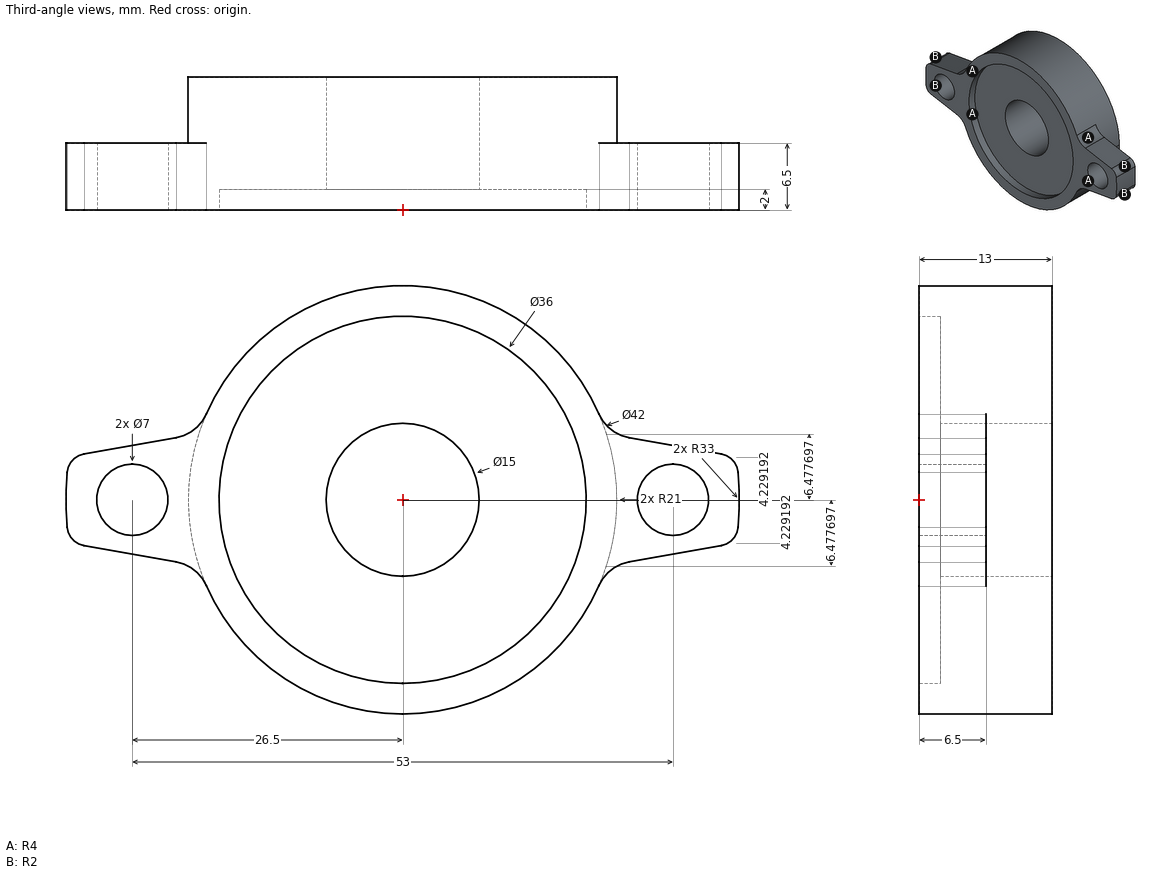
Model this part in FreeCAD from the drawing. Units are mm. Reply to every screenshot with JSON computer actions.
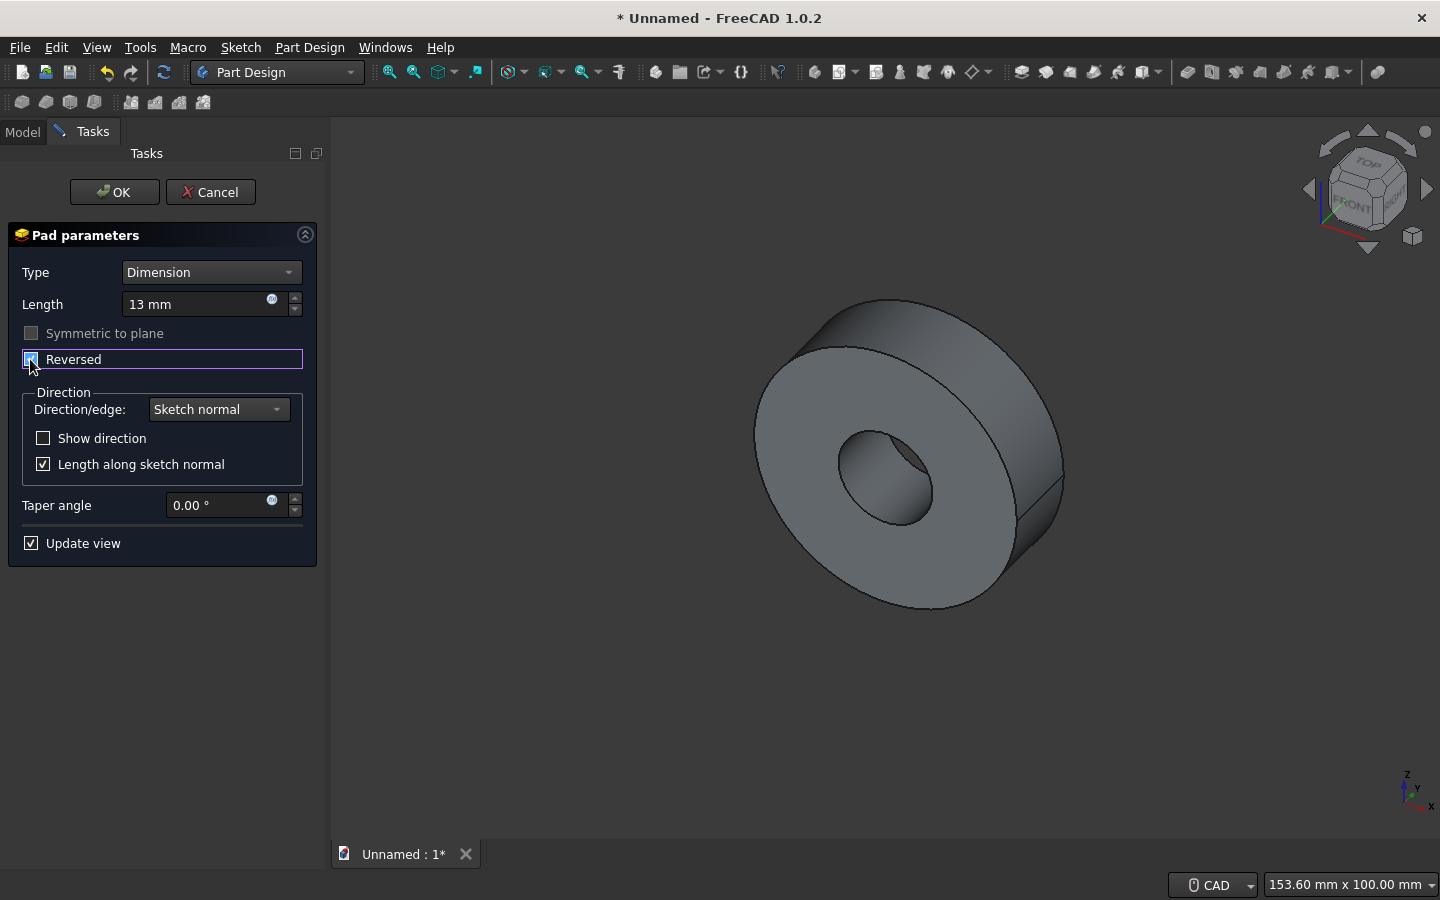
{"action": "left_click", "coordinate": [115, 192]}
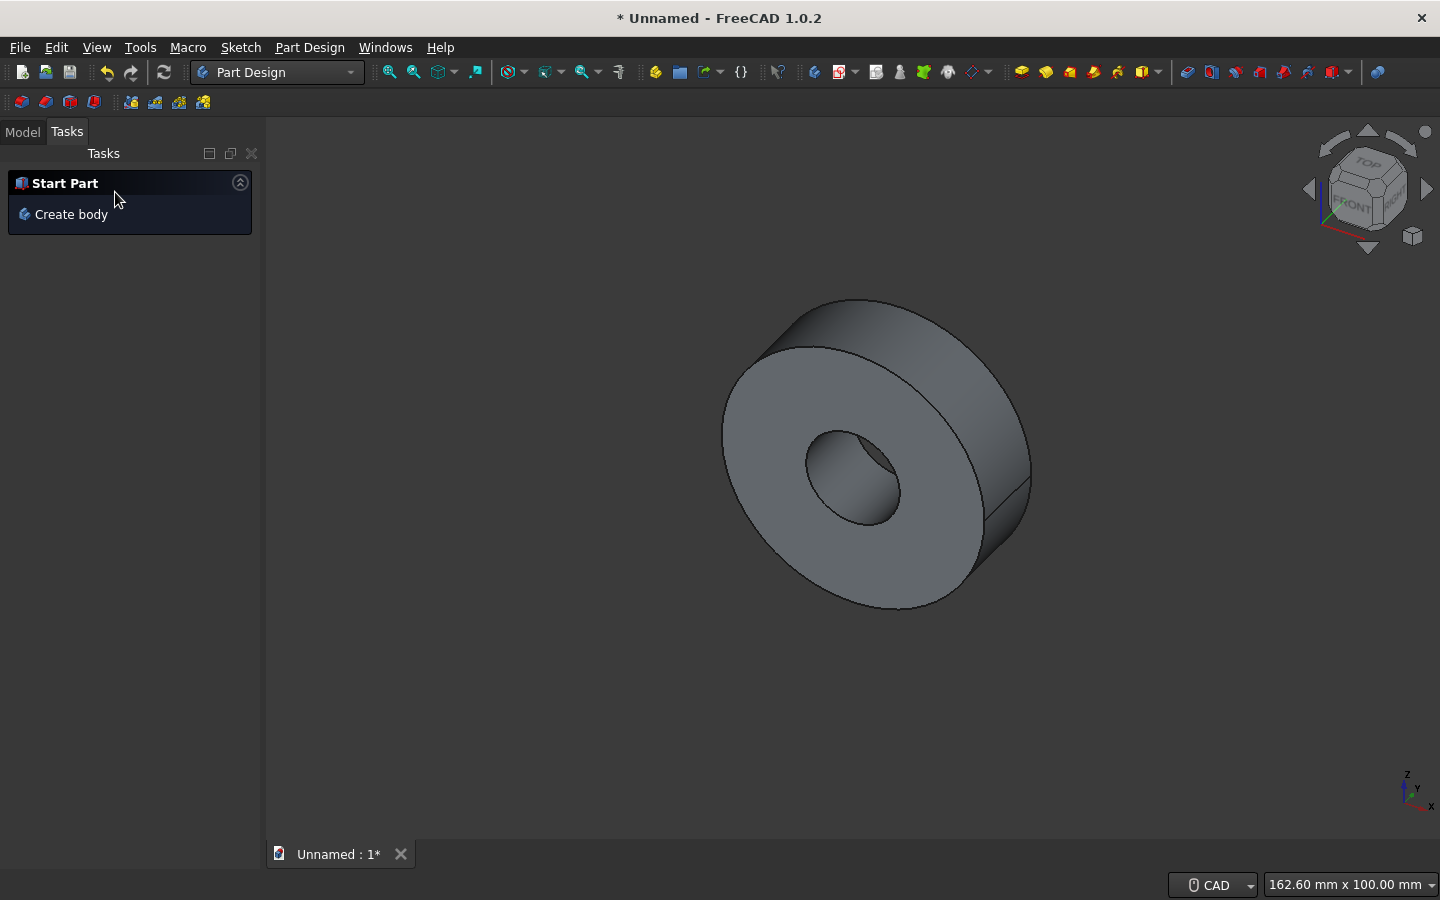
{"action": "left_click", "coordinate": [815, 536]}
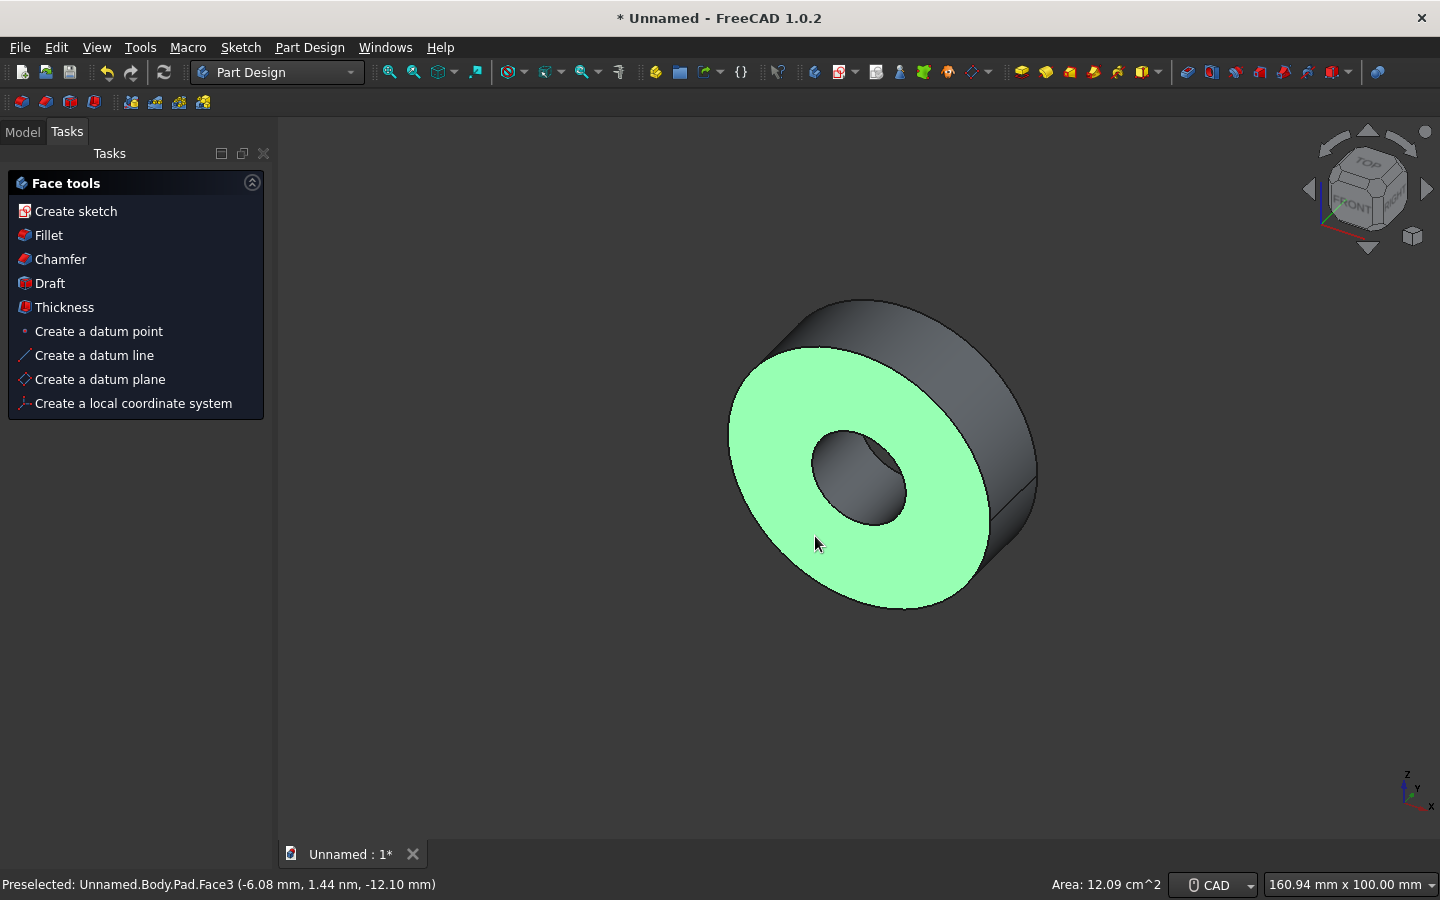
{"action": "left_click", "coordinate": [840, 72]}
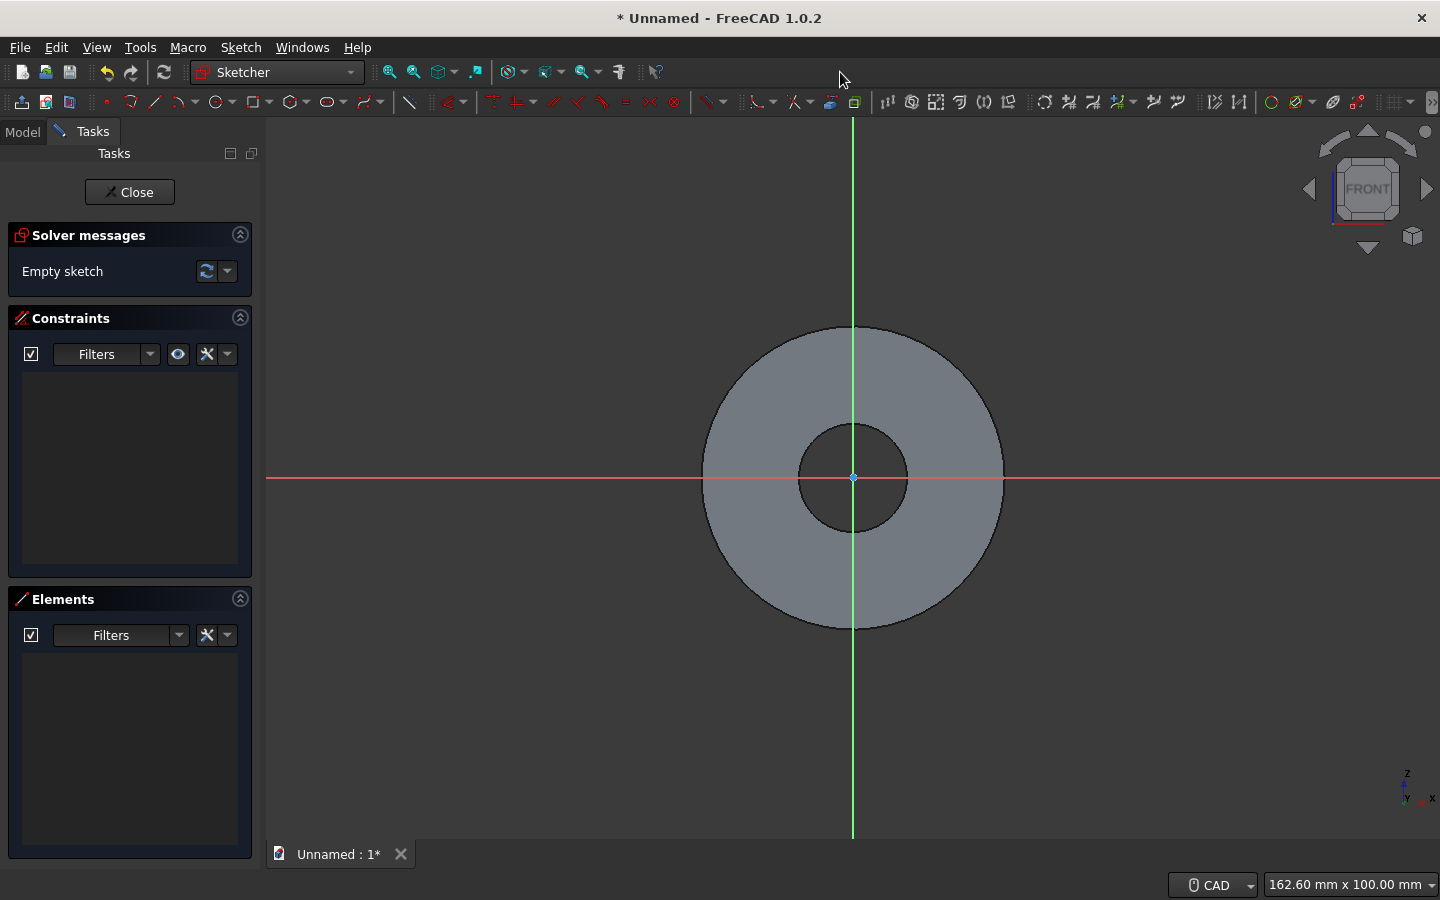
{"action": "scroll", "coordinate": [992, 478], "scroll_direction": "up", "scroll_amount": 2}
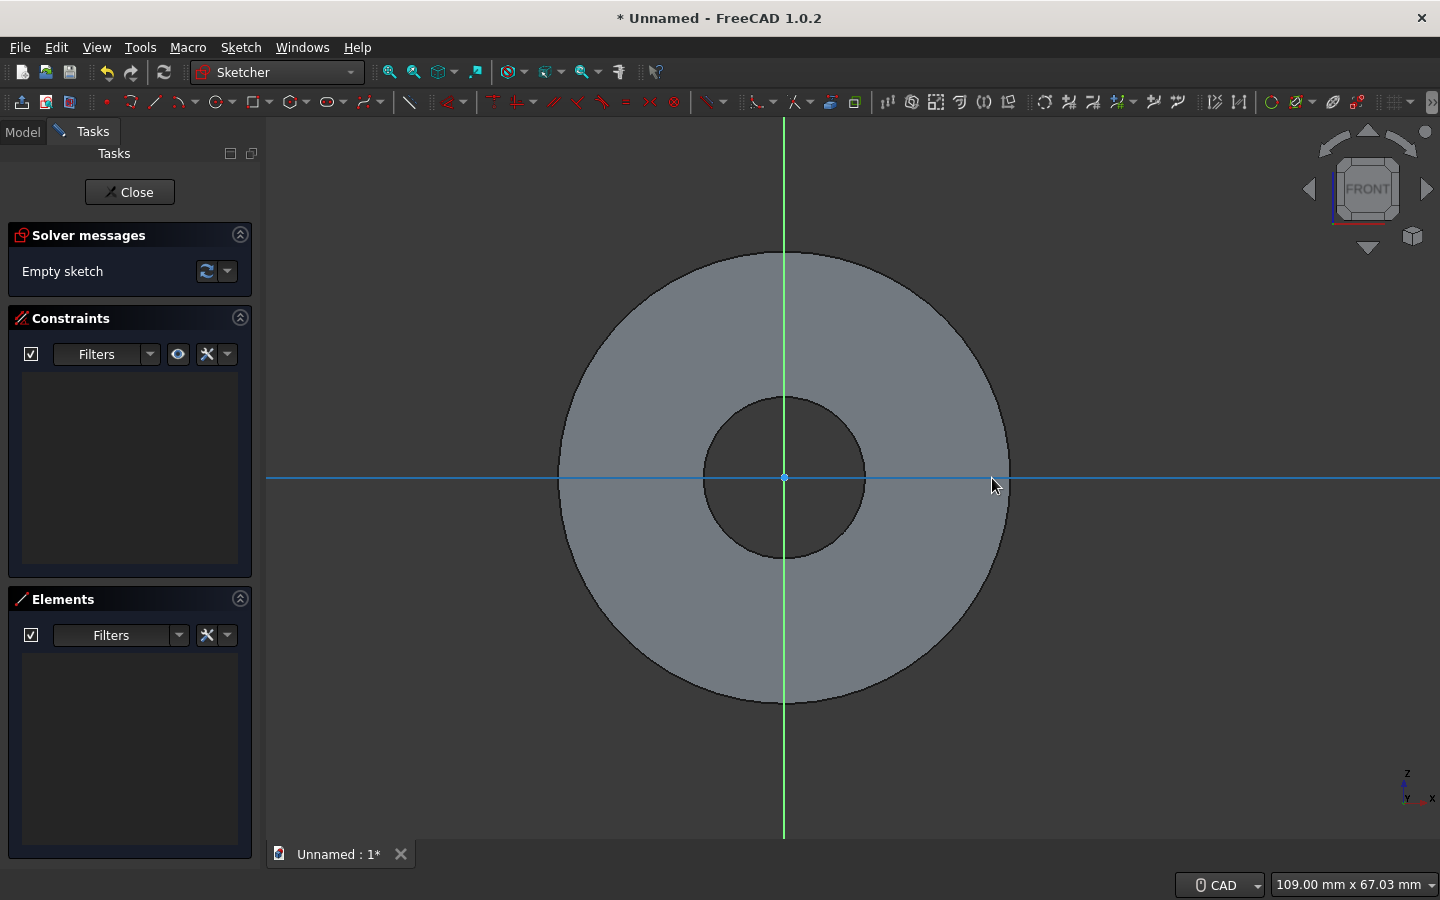
{"action": "left_click", "coordinate": [156, 102]}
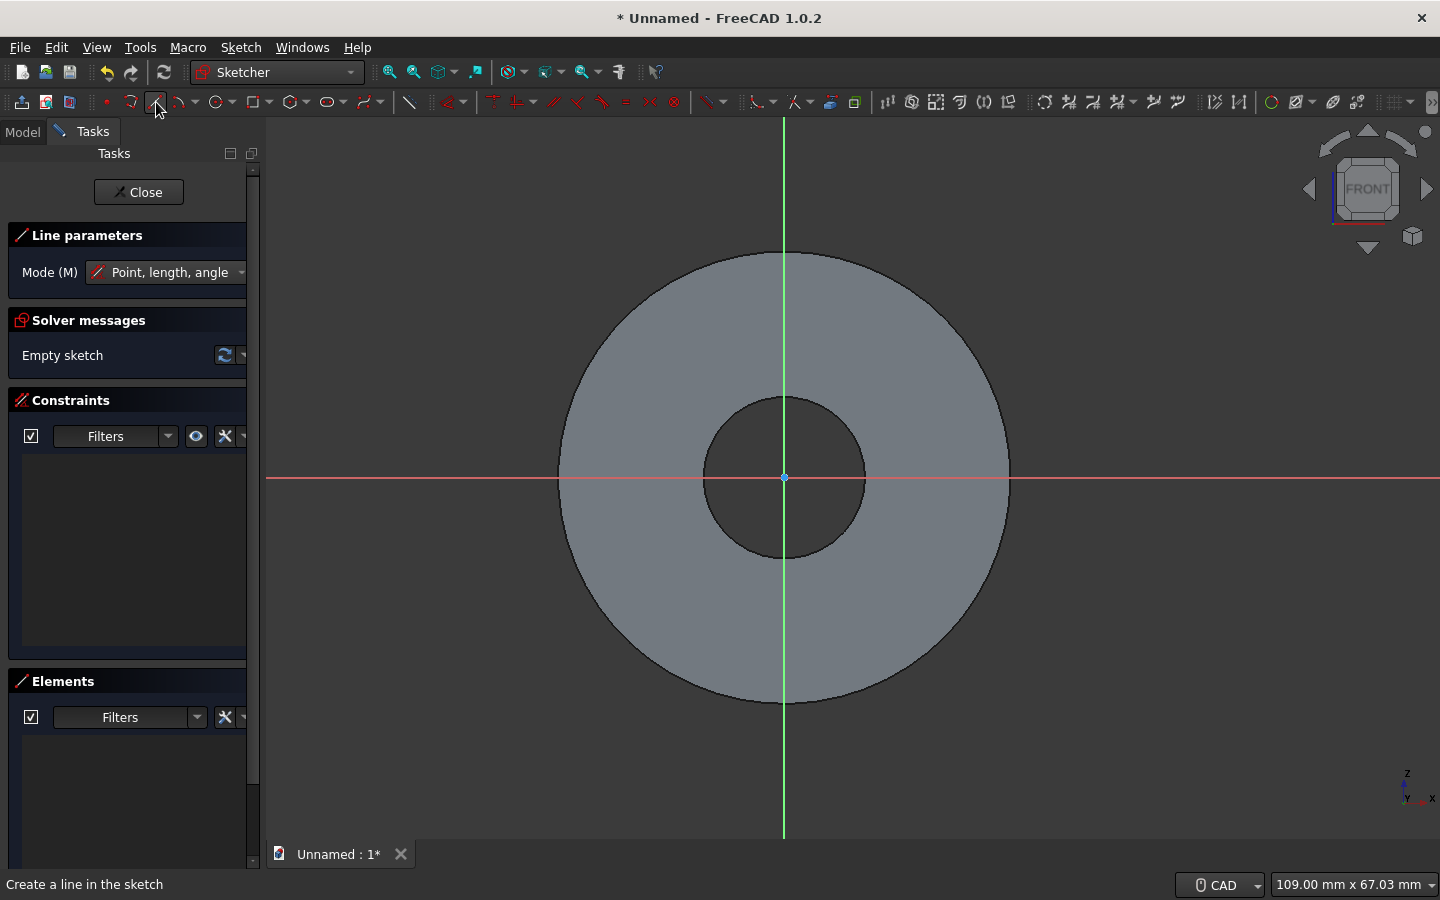
{"action": "left_click", "coordinate": [1137, 432]}
{"action": "left_click", "coordinate": [999, 408]}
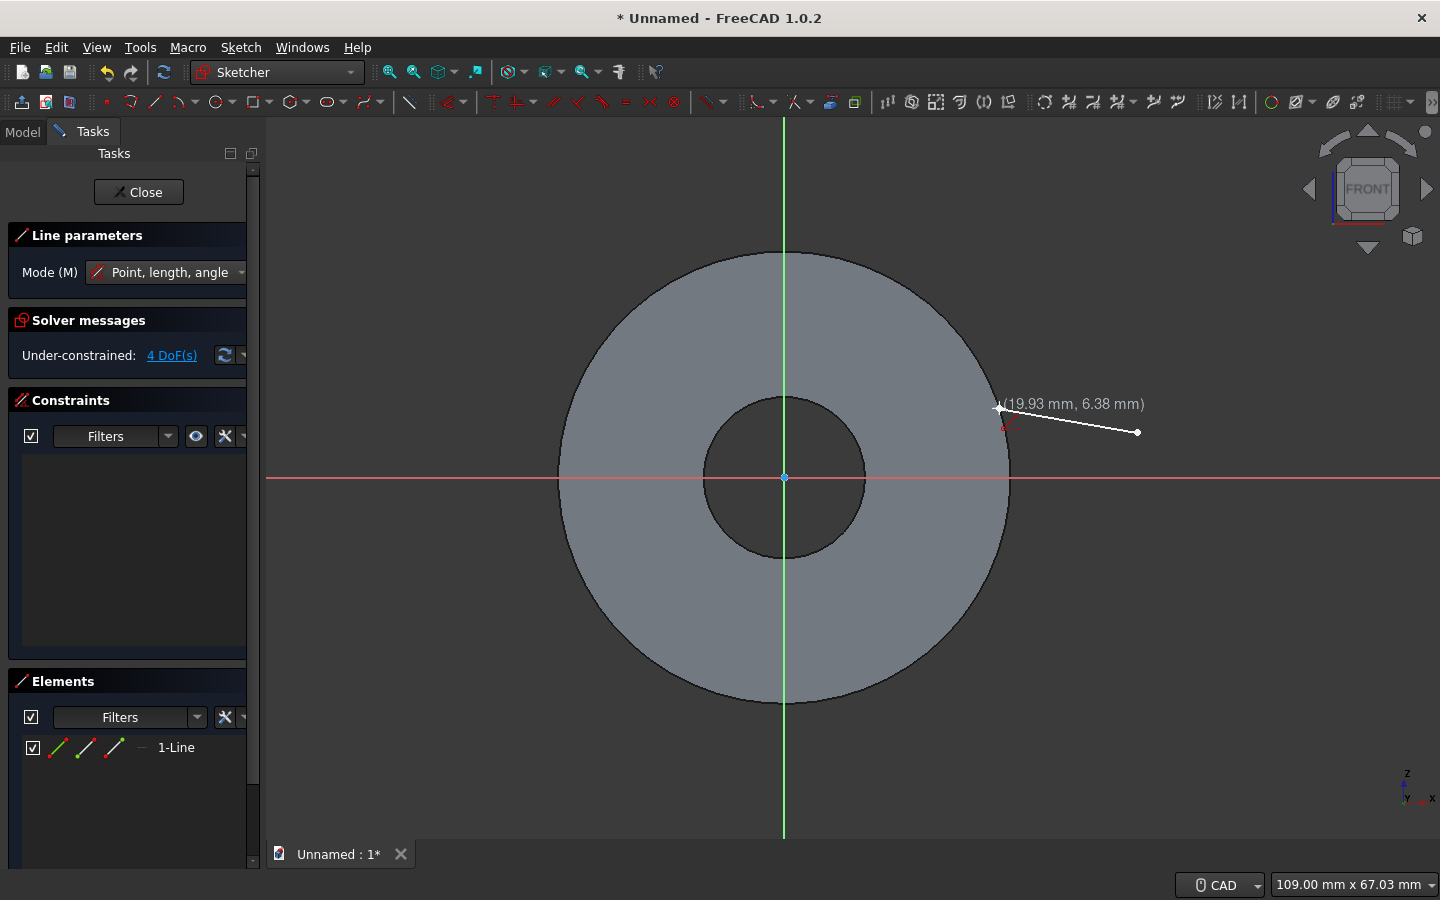
{"action": "left_click", "coordinate": [999, 548]}
{"action": "left_click", "coordinate": [1137, 523]}